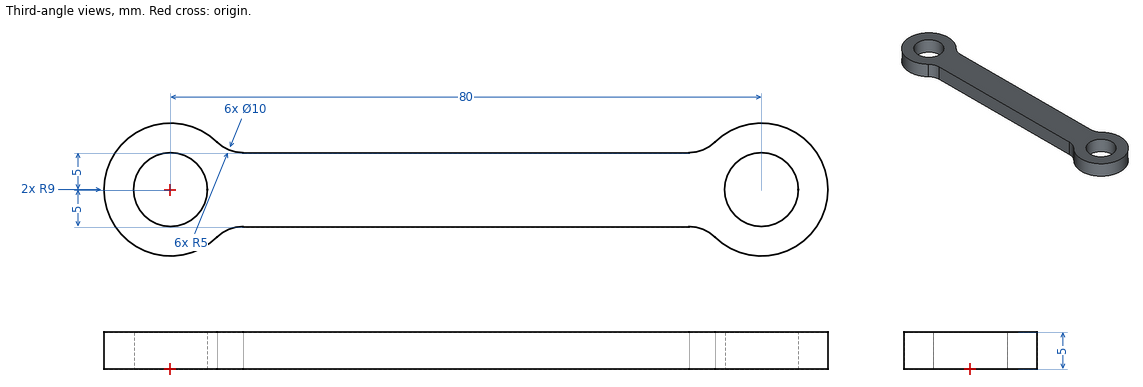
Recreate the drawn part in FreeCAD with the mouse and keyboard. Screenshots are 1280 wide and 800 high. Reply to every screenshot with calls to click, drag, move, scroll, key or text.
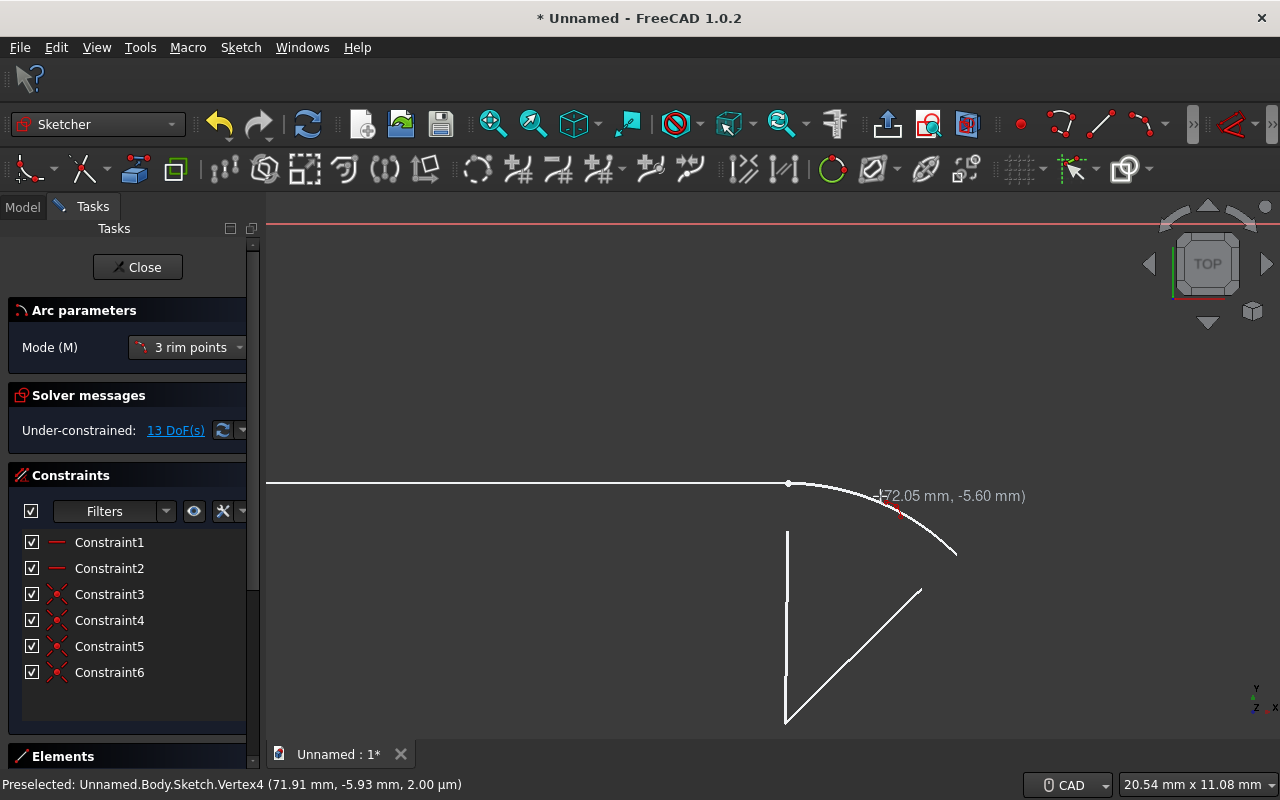
click(877, 489)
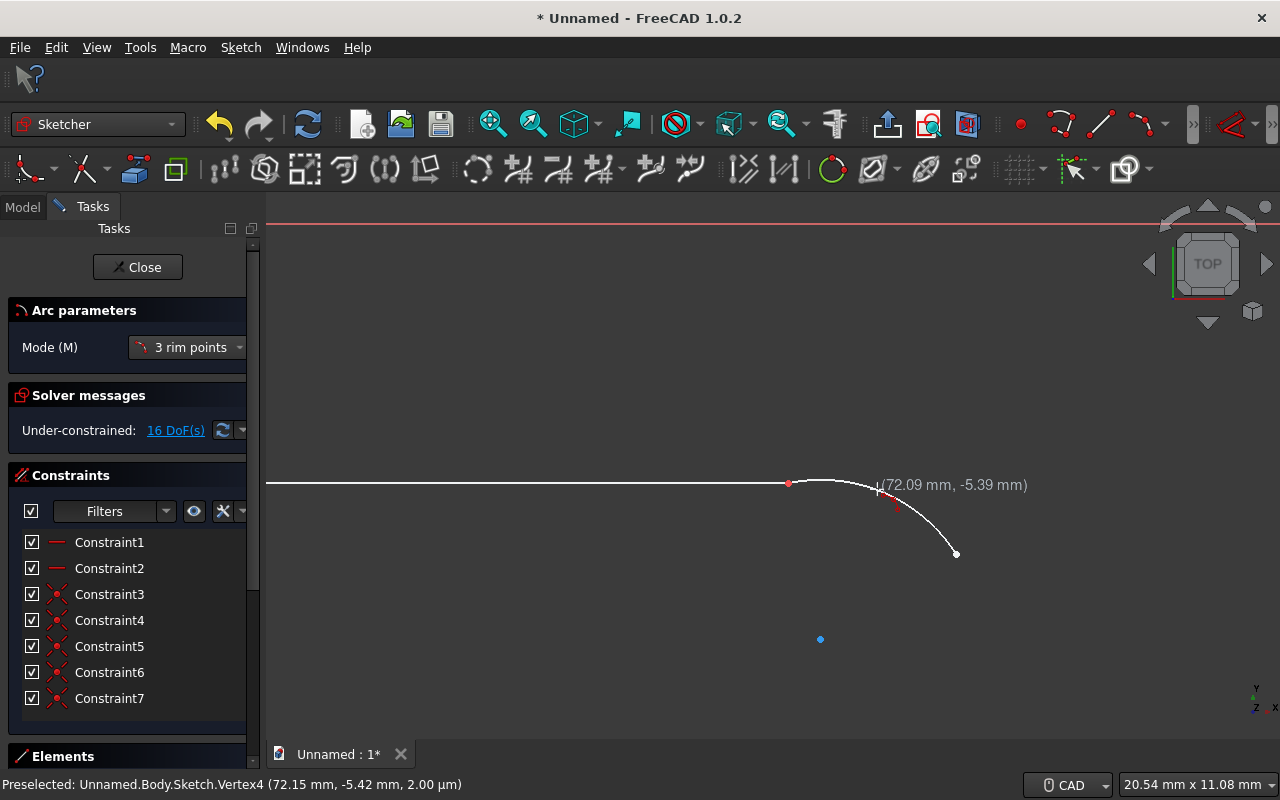
scroll(880, 496, down, 11)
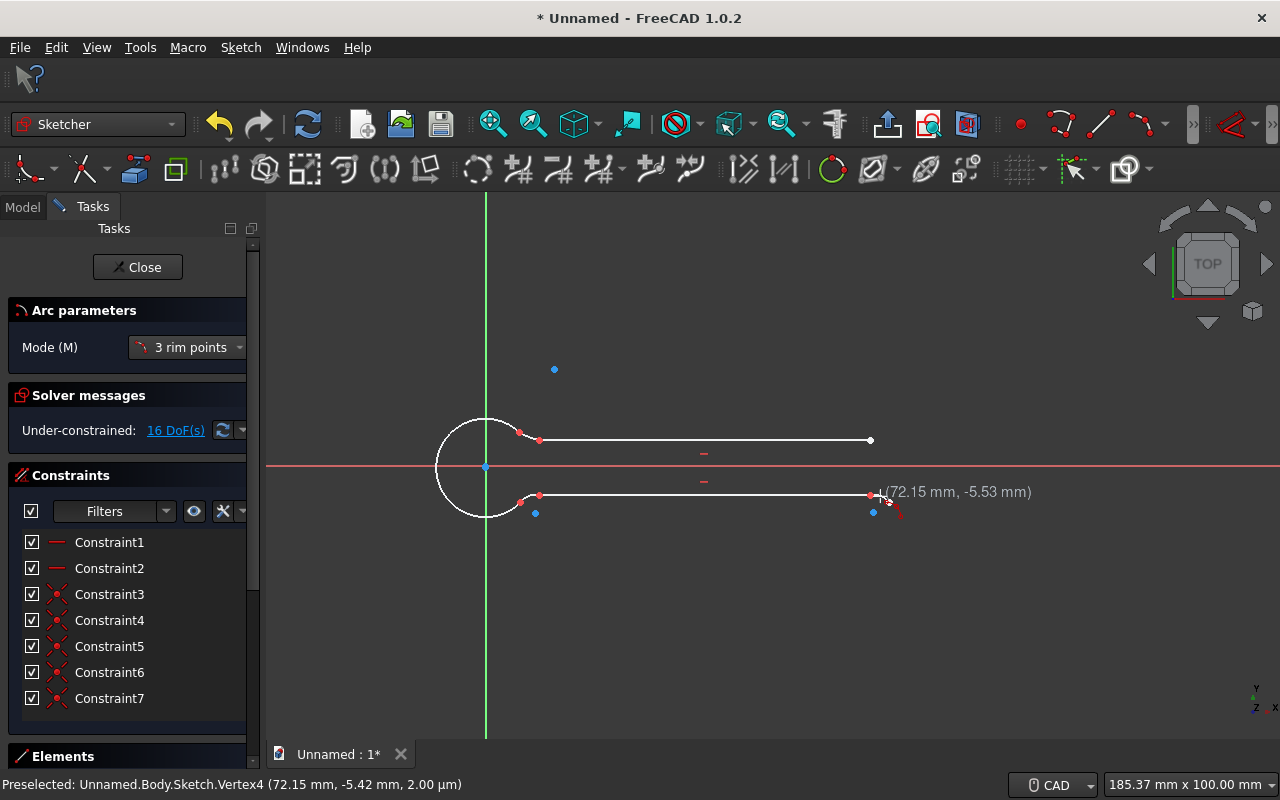
click(889, 503)
click(889, 431)
click(967, 489)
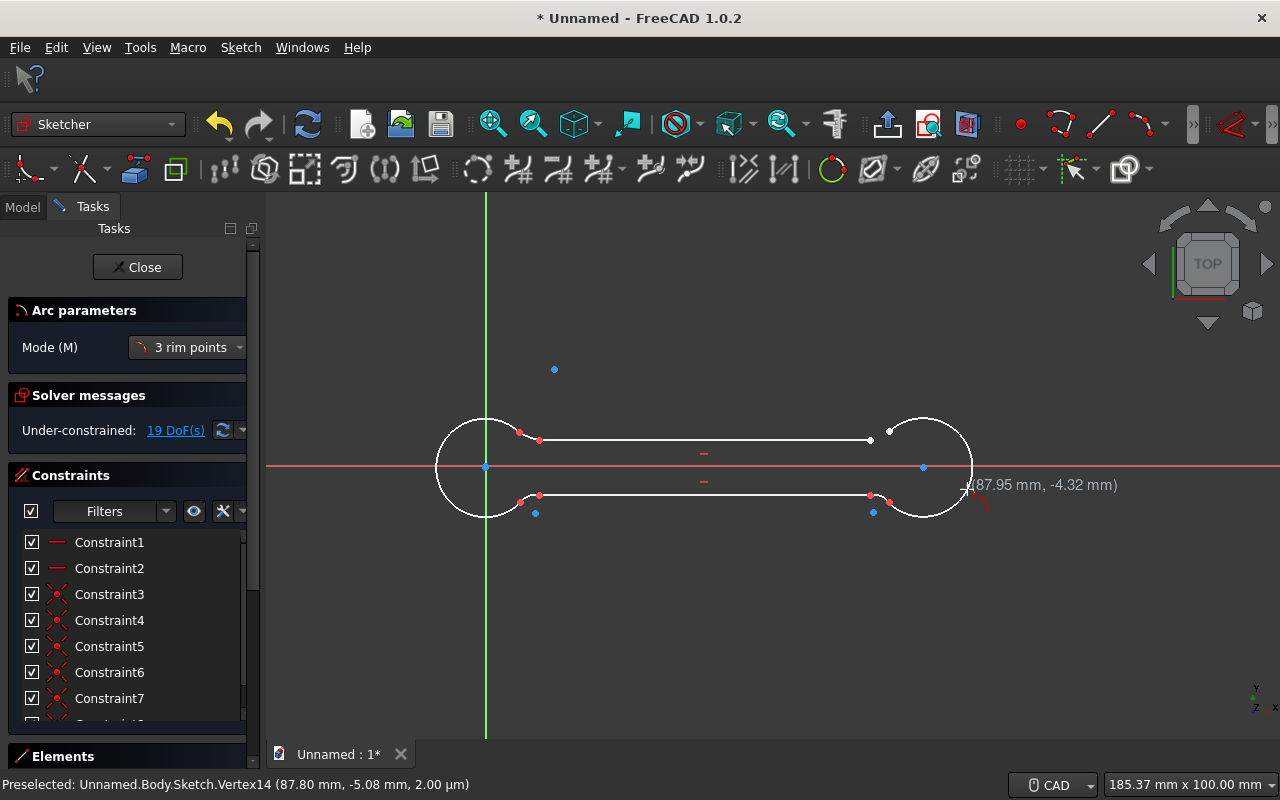
click(889, 432)
click(870, 440)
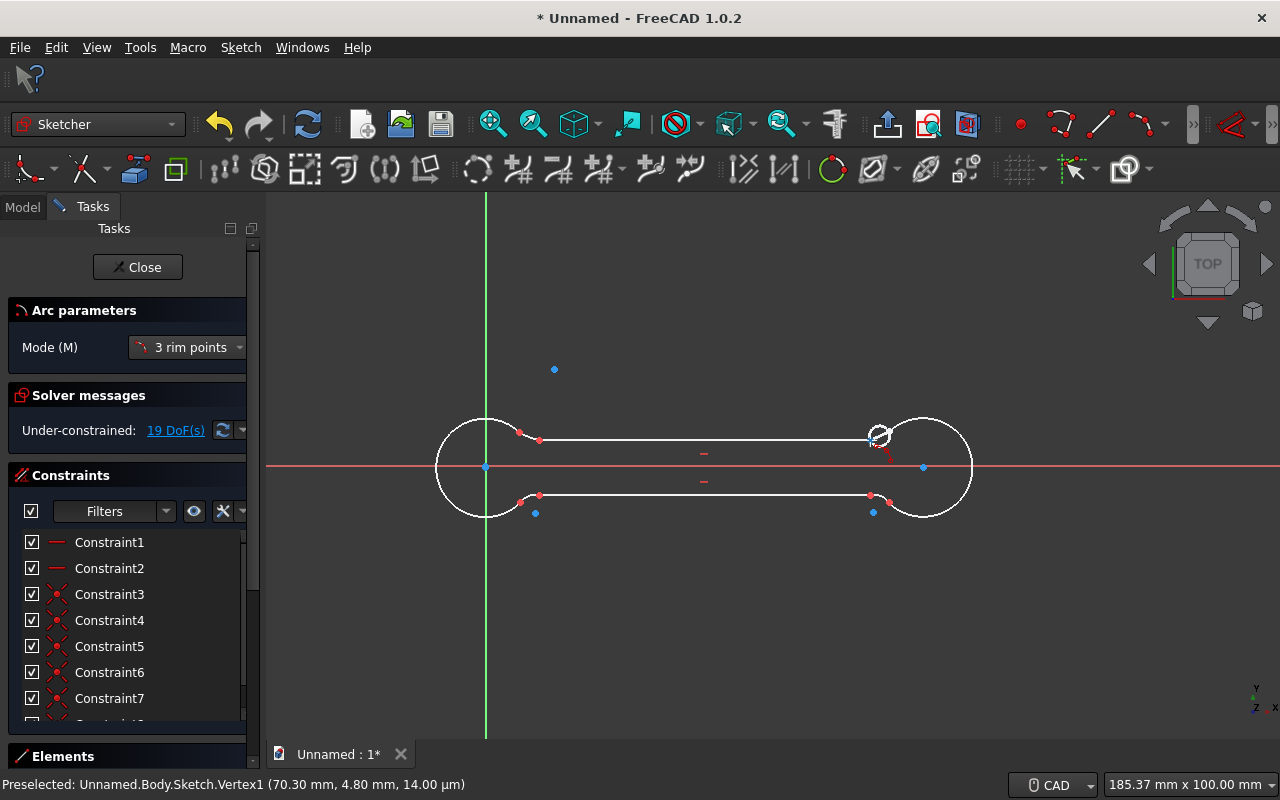
scroll(880, 437, up, 11)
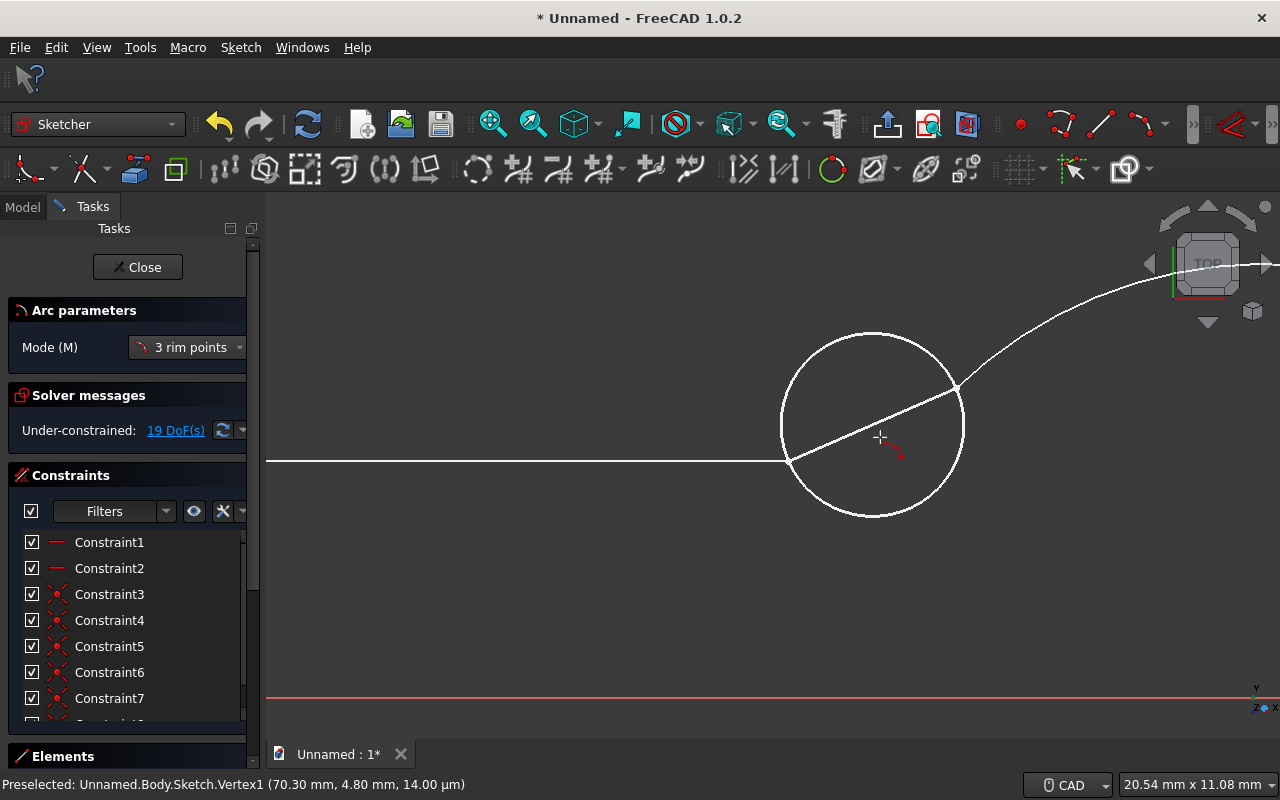
click(877, 433)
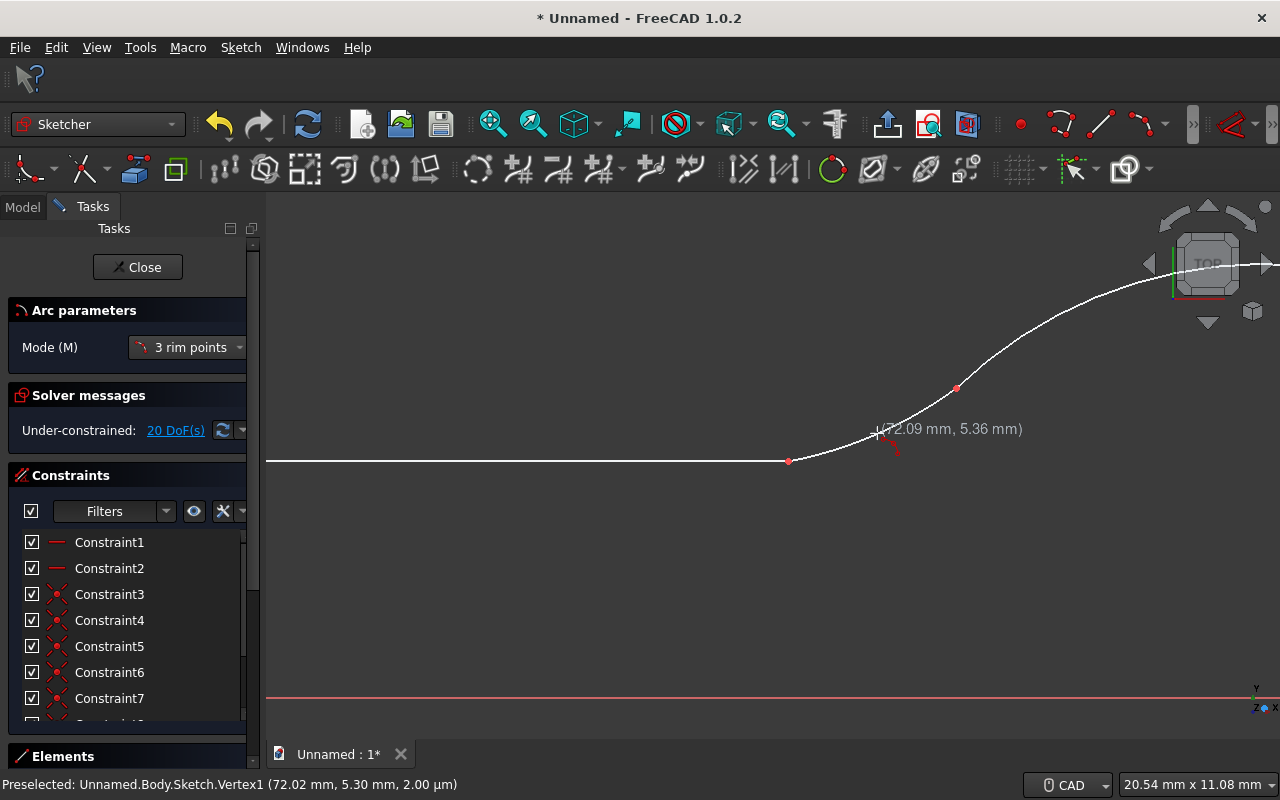
key(g)
key(c)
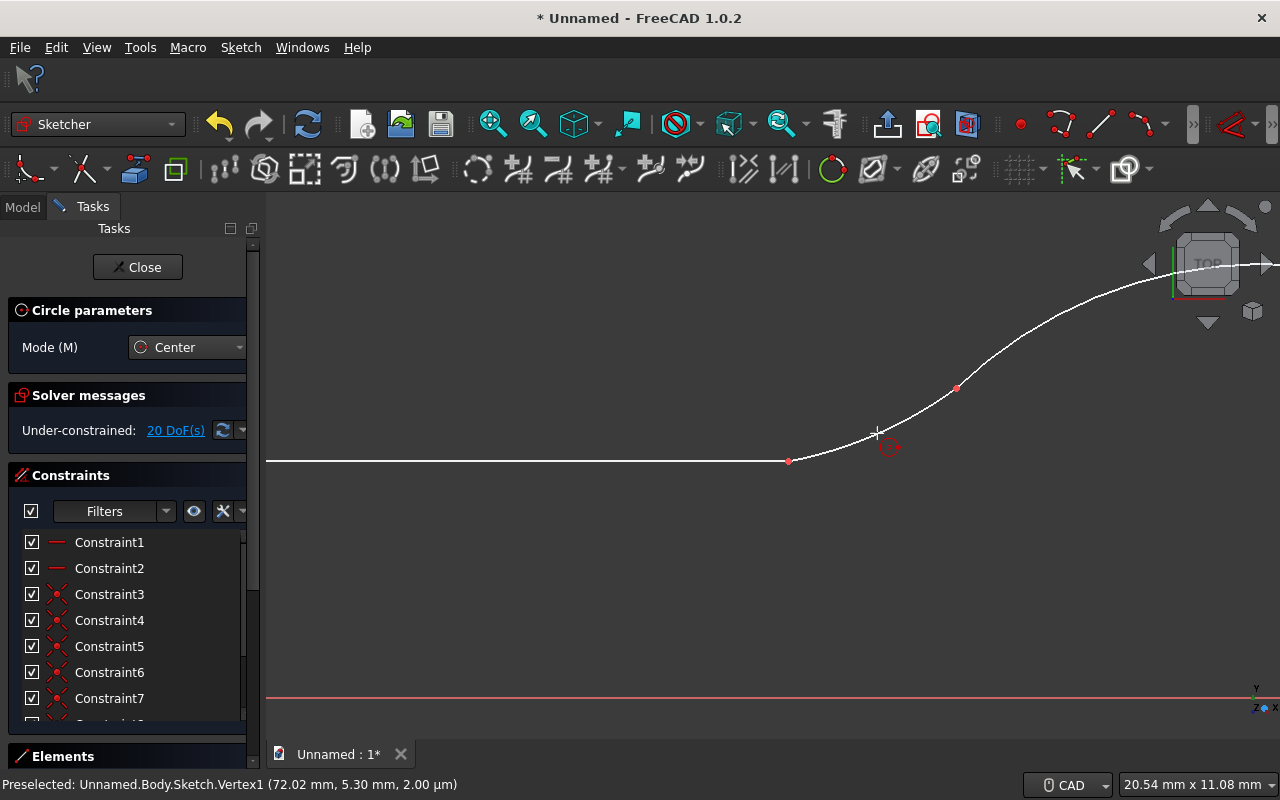
scroll(880, 436, down, 11)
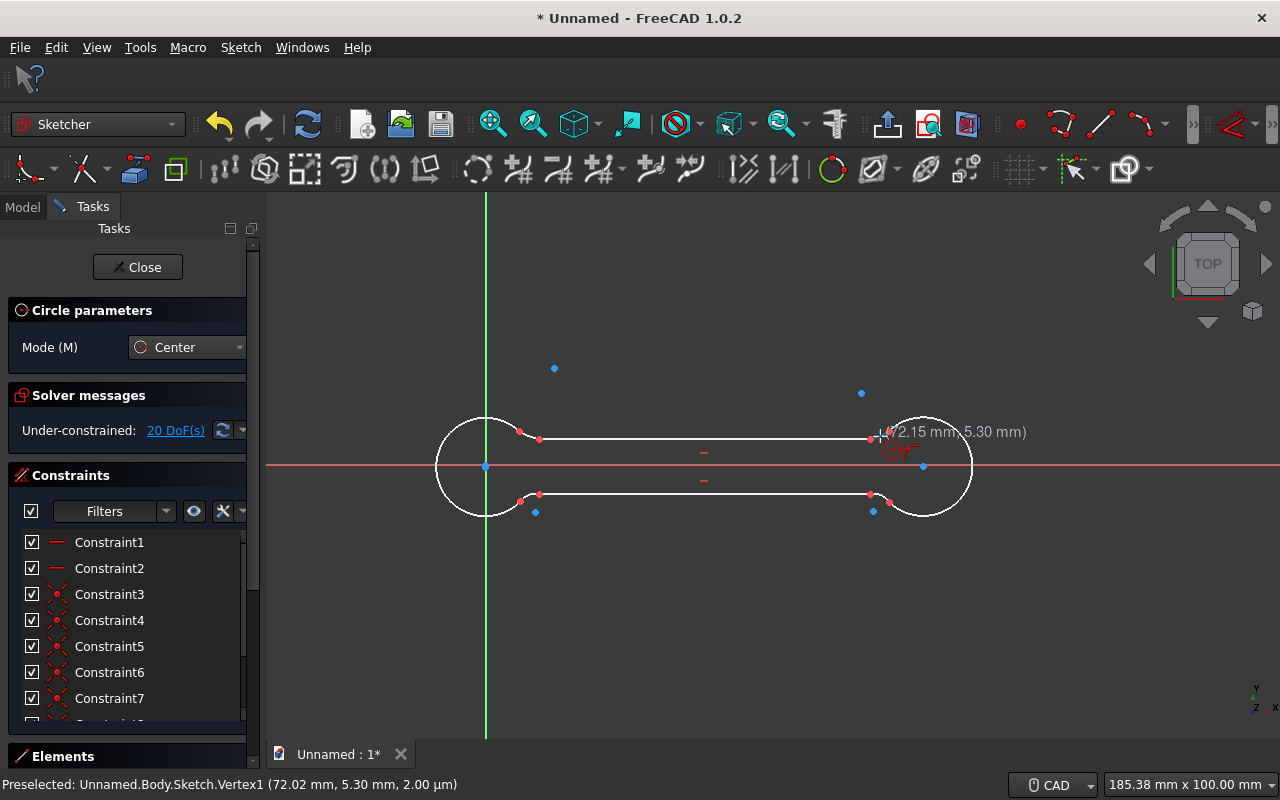
click(923, 465)
move(943, 446)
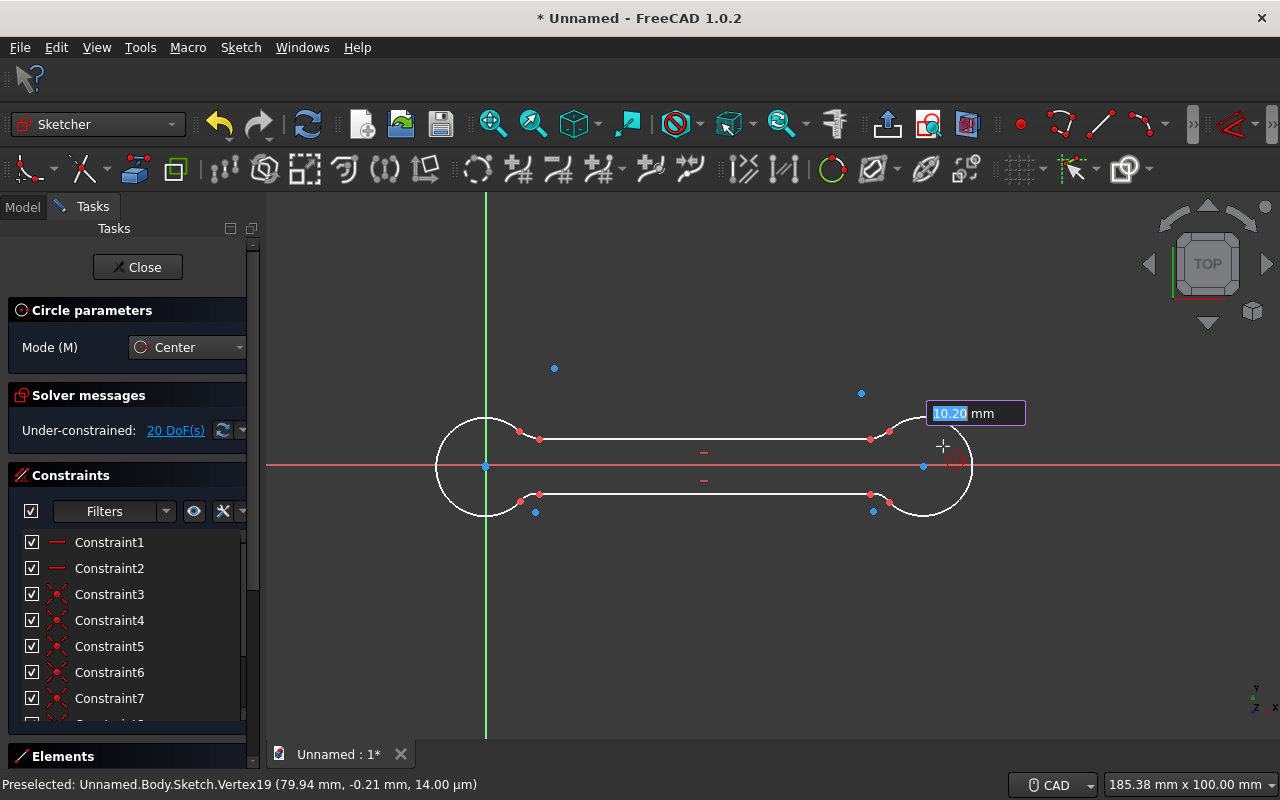
text(10)
key(Return)